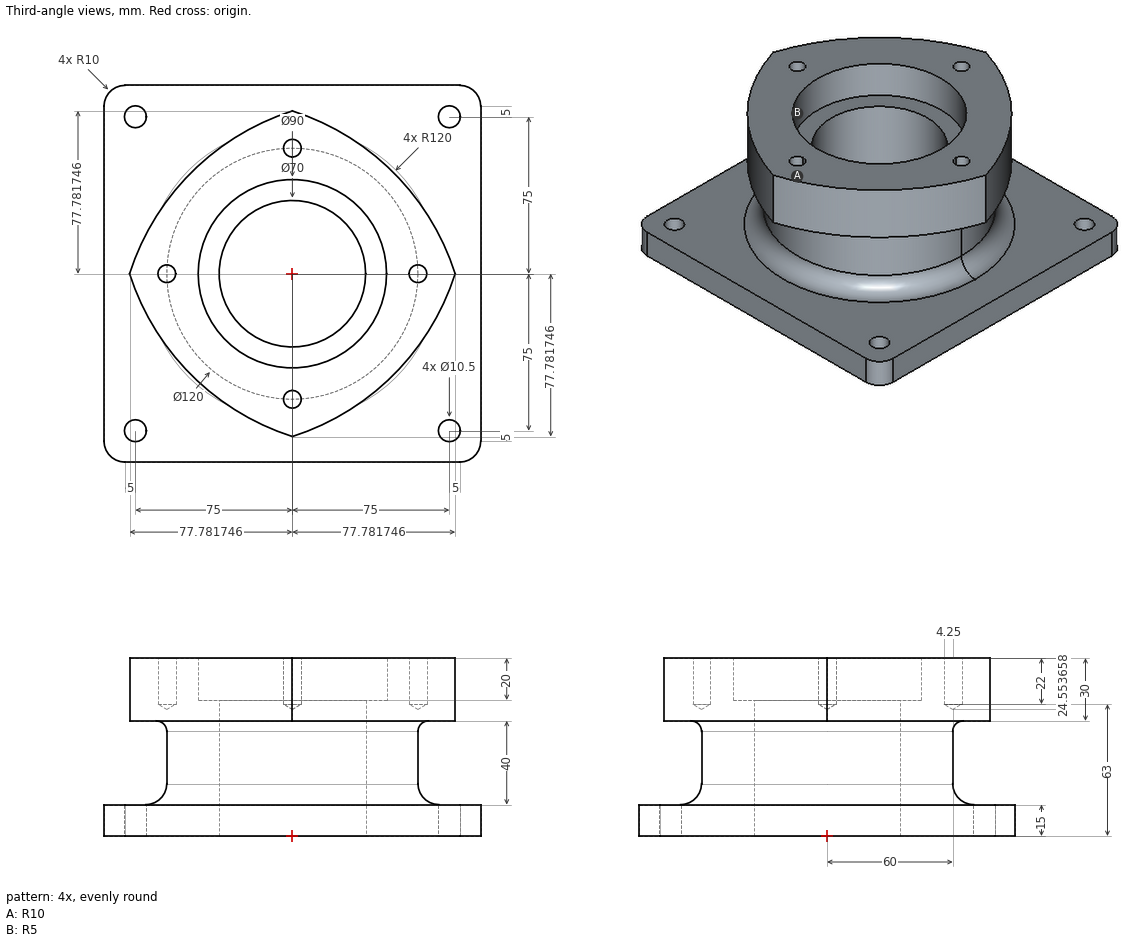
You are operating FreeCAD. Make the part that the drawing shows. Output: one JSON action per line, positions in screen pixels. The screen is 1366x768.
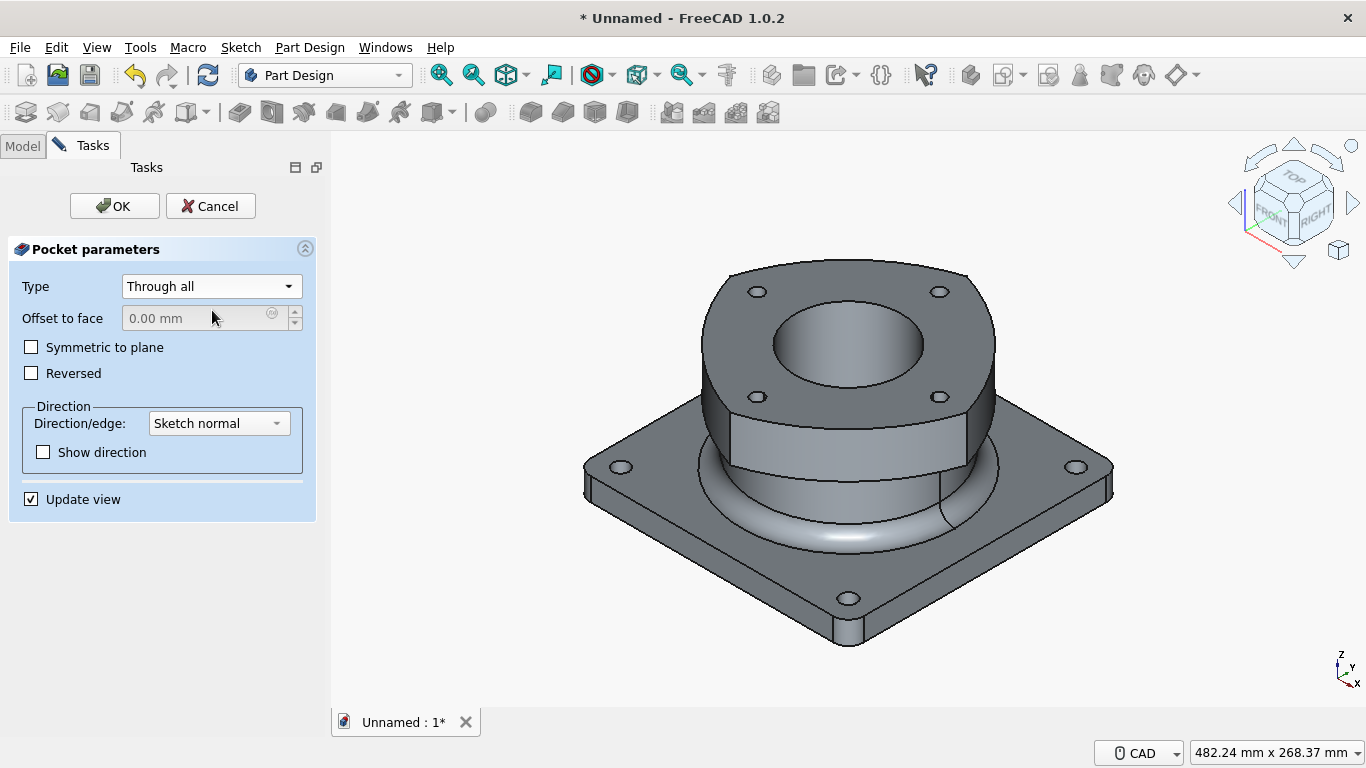
{"action": "left_click", "coordinate": [115, 206]}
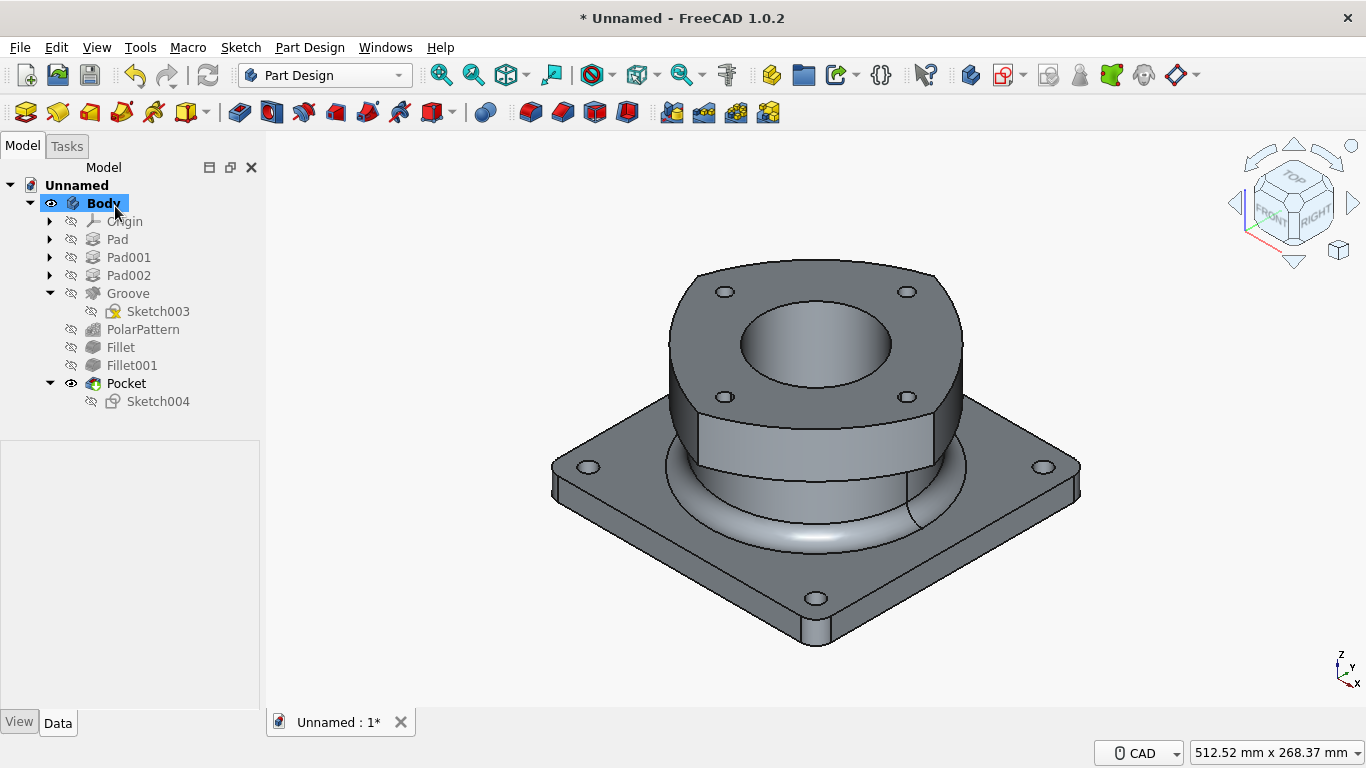
{"action": "left_click", "coordinate": [715, 363]}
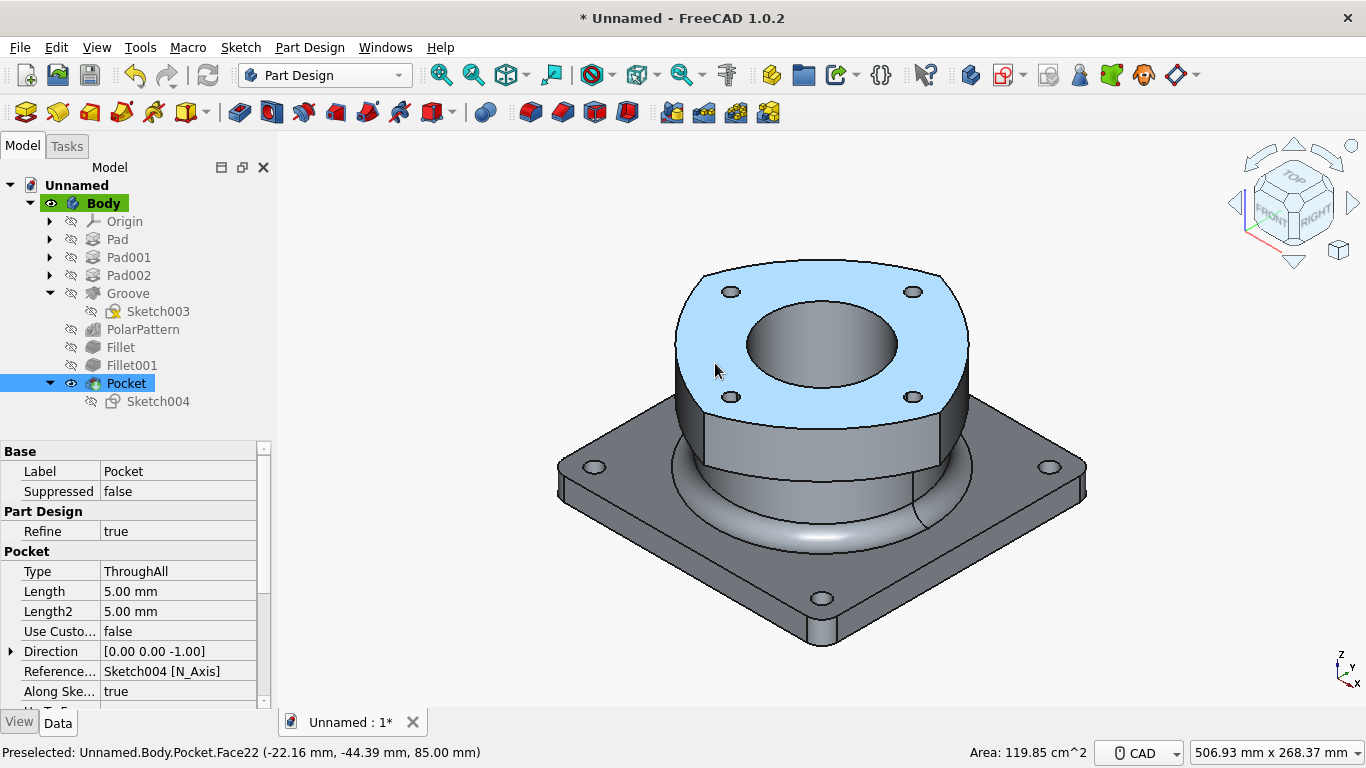
{"action": "left_click", "coordinate": [1004, 76]}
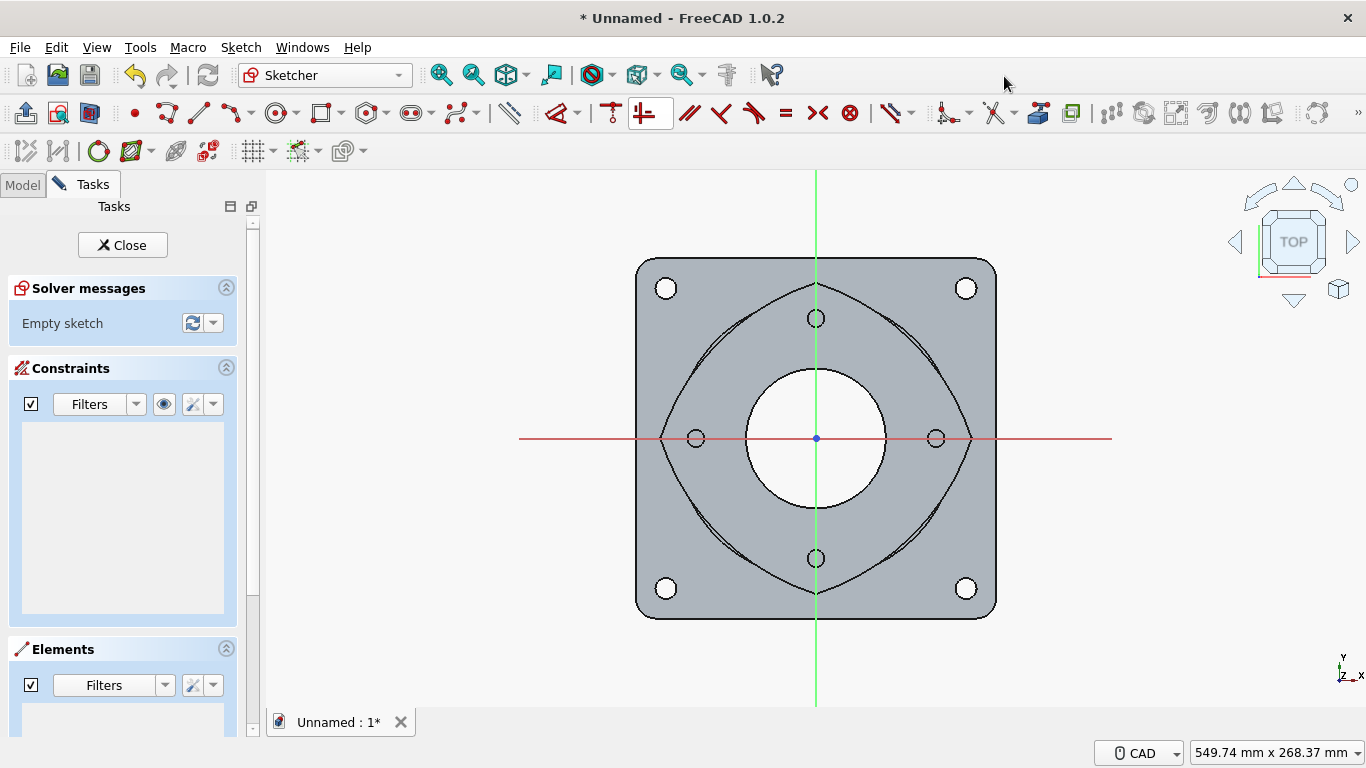
{"action": "scroll", "coordinate": [899, 438], "scroll_direction": "up", "scroll_amount": 3}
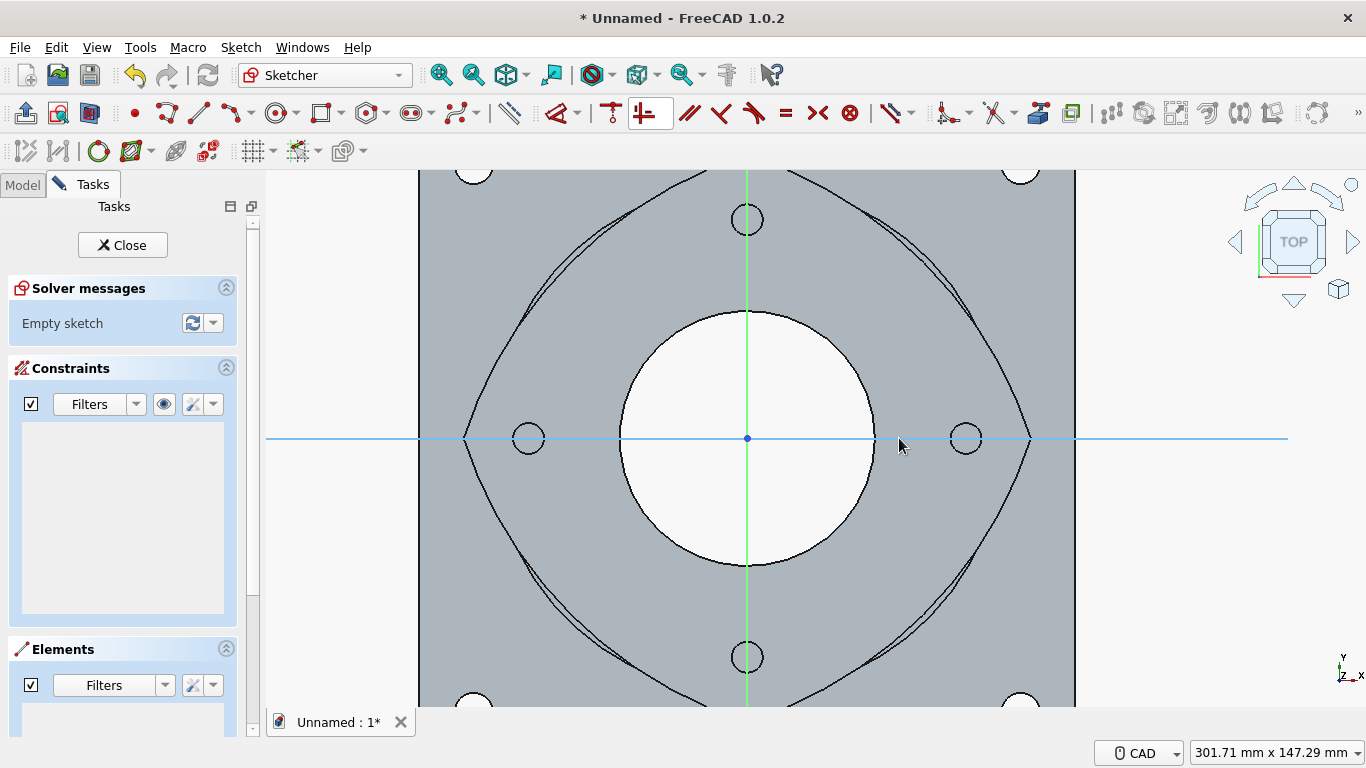
{"action": "left_click", "coordinate": [276, 114]}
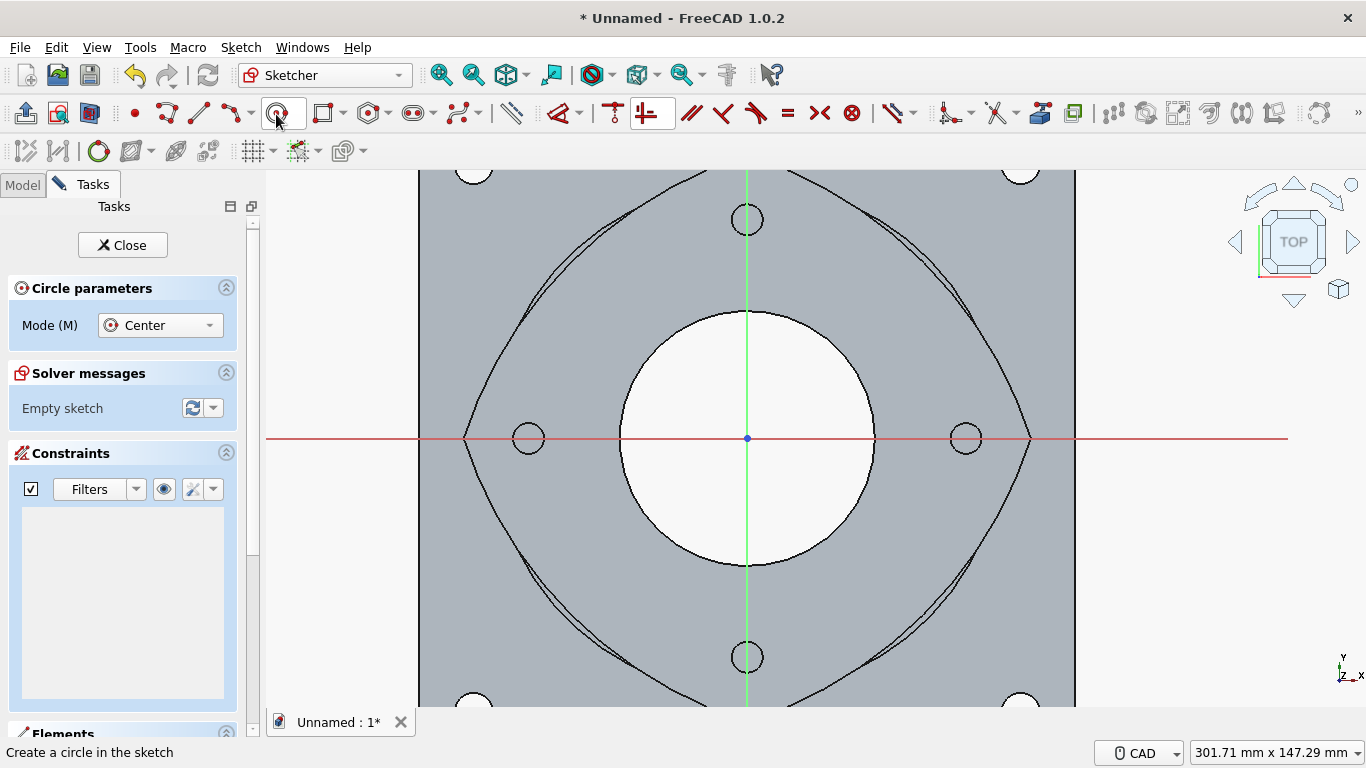
{"action": "left_click", "coordinate": [747, 438]}
{"action": "mouse_move", "coordinate": [863, 322]}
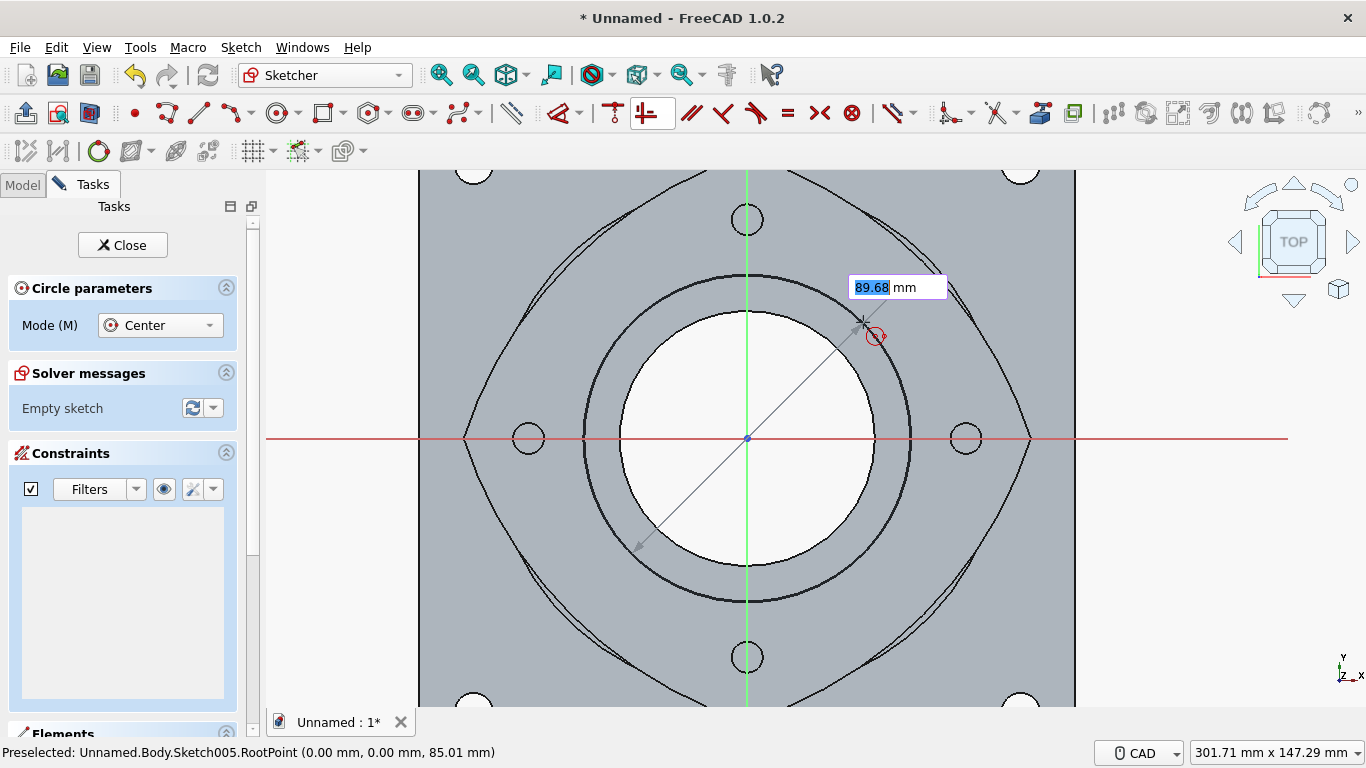
{"action": "type", "text": "90"}
{"action": "key", "text": "Return"}
{"action": "key", "text": "Escape"}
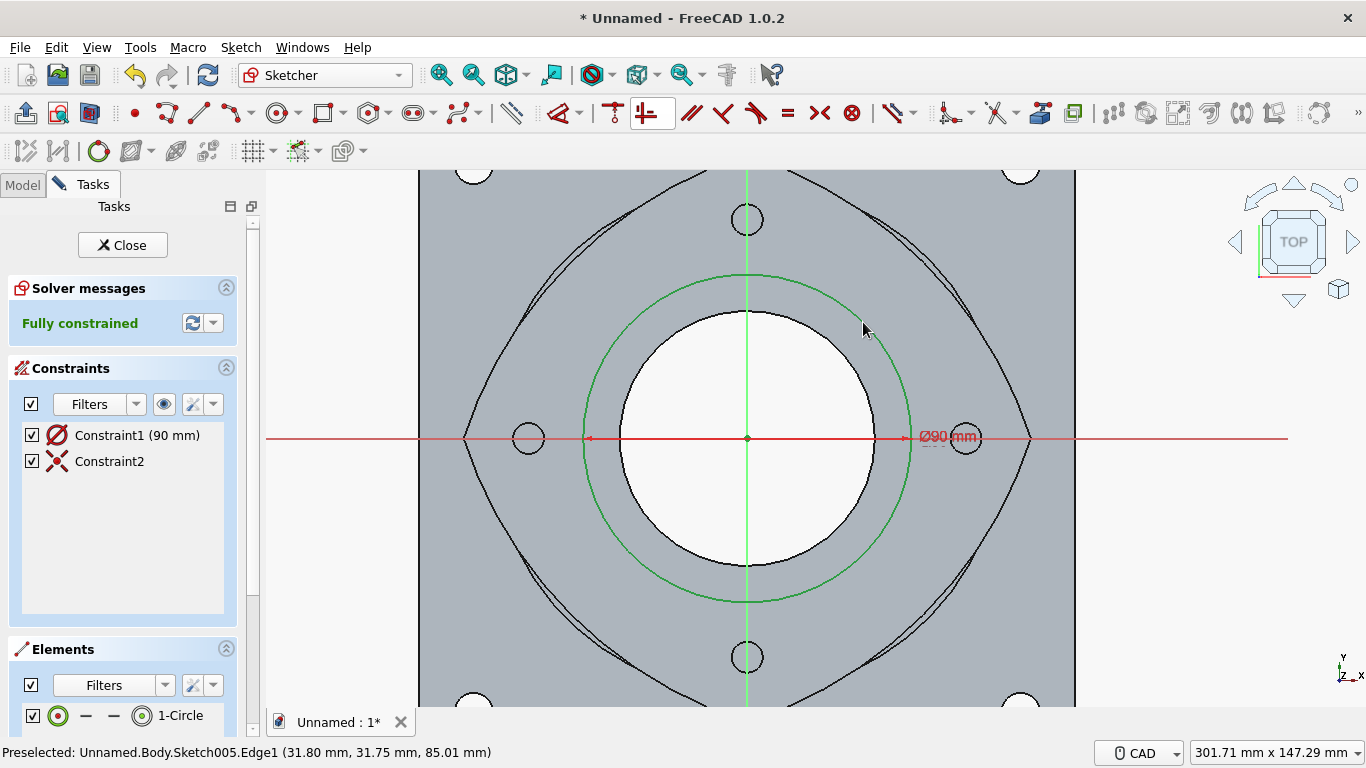
{"action": "left_click", "coordinate": [123, 245]}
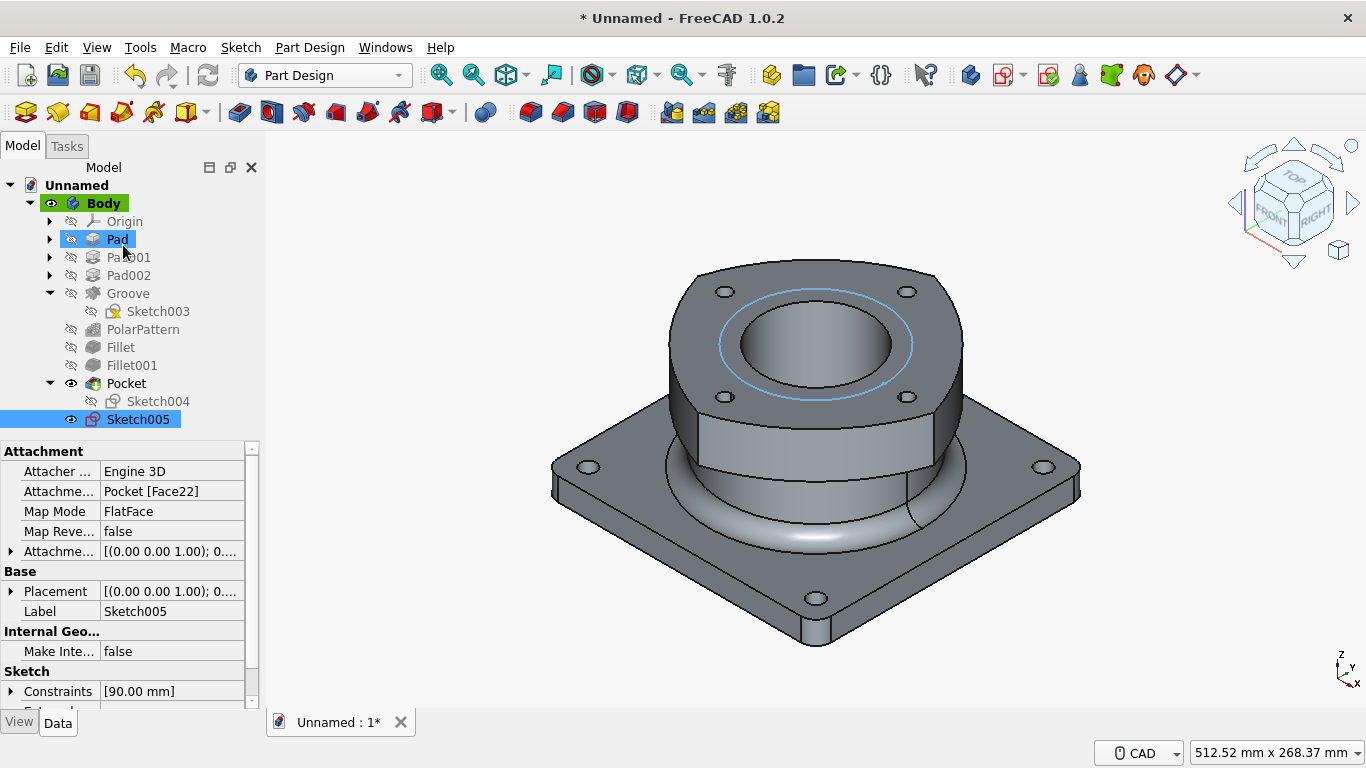
{"action": "left_click", "coordinate": [240, 112]}